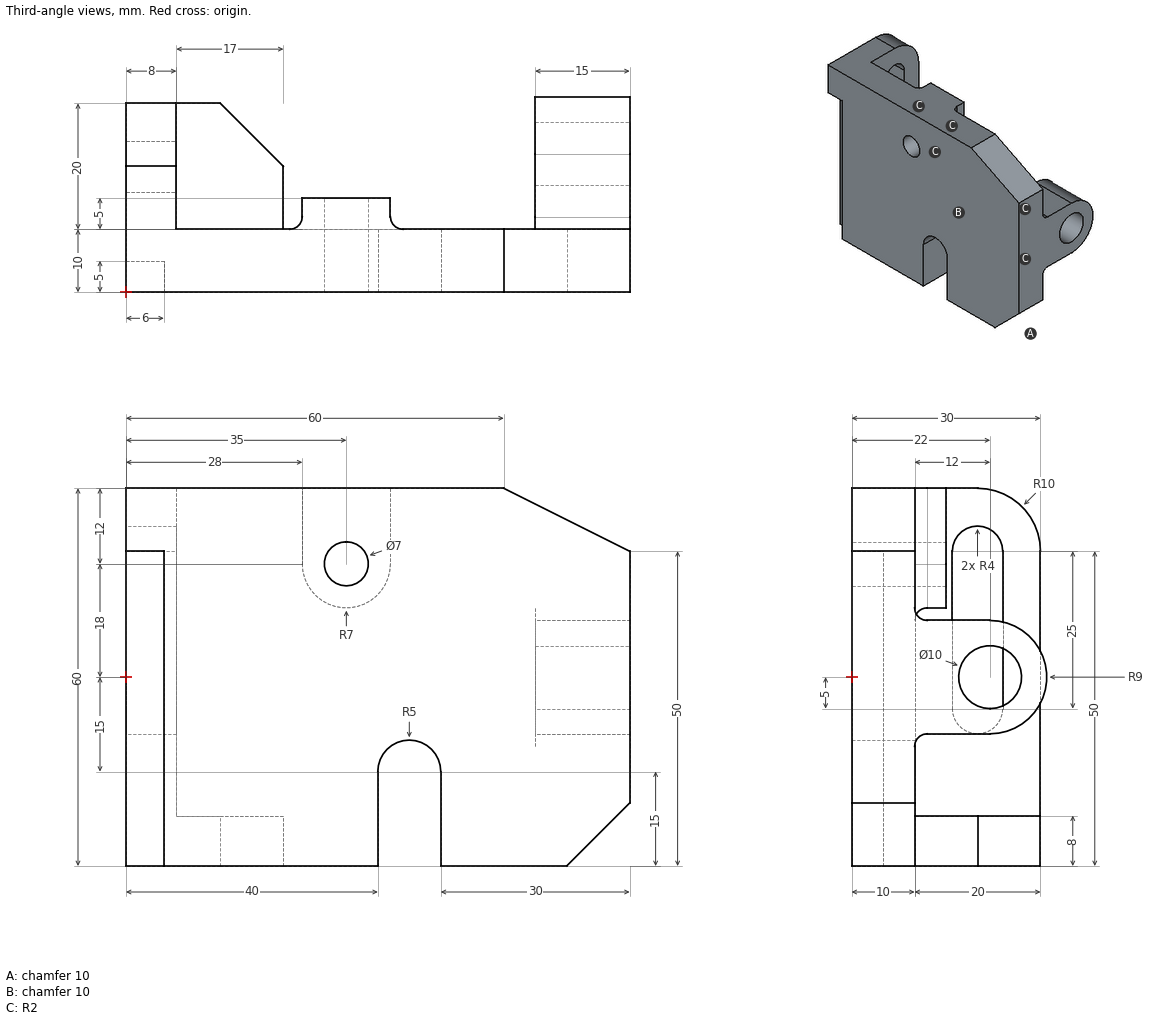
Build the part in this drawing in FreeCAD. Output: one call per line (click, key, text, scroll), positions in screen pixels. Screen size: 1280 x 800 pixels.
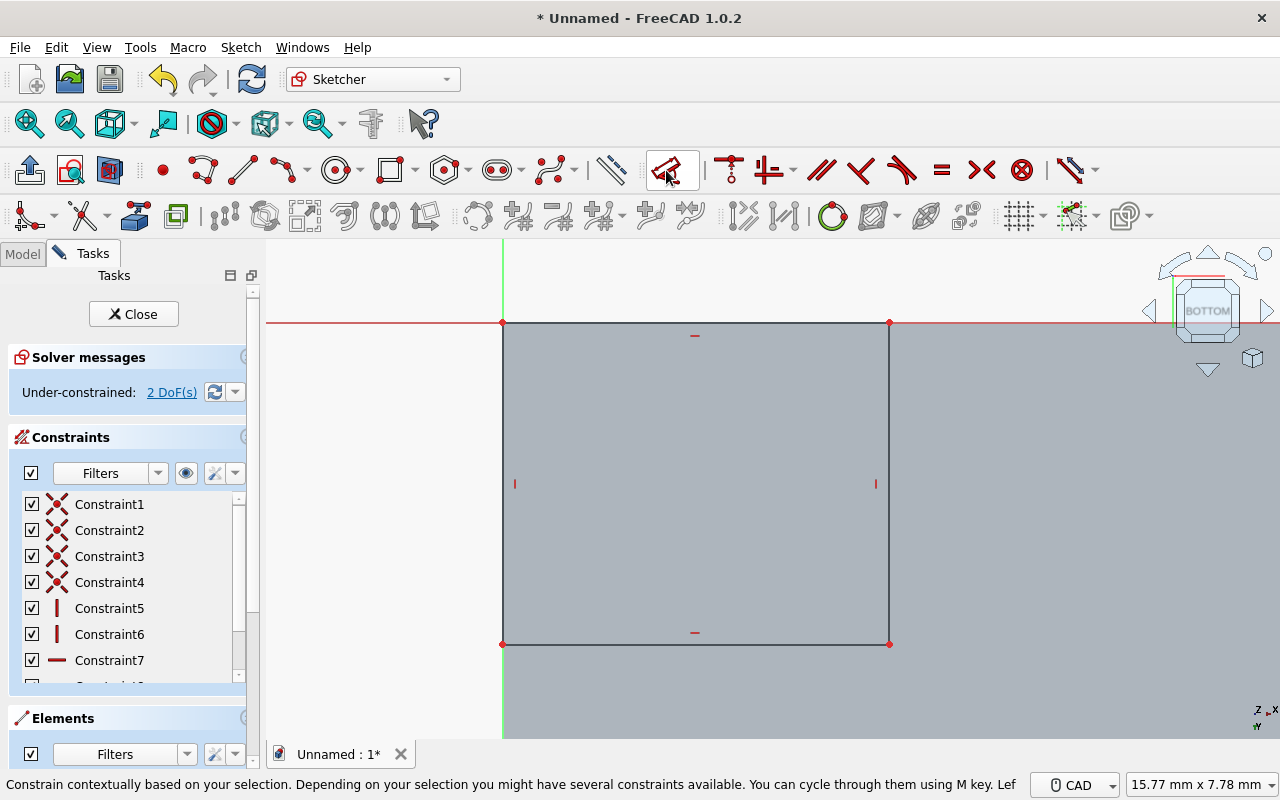
click(503, 419)
click(469, 484)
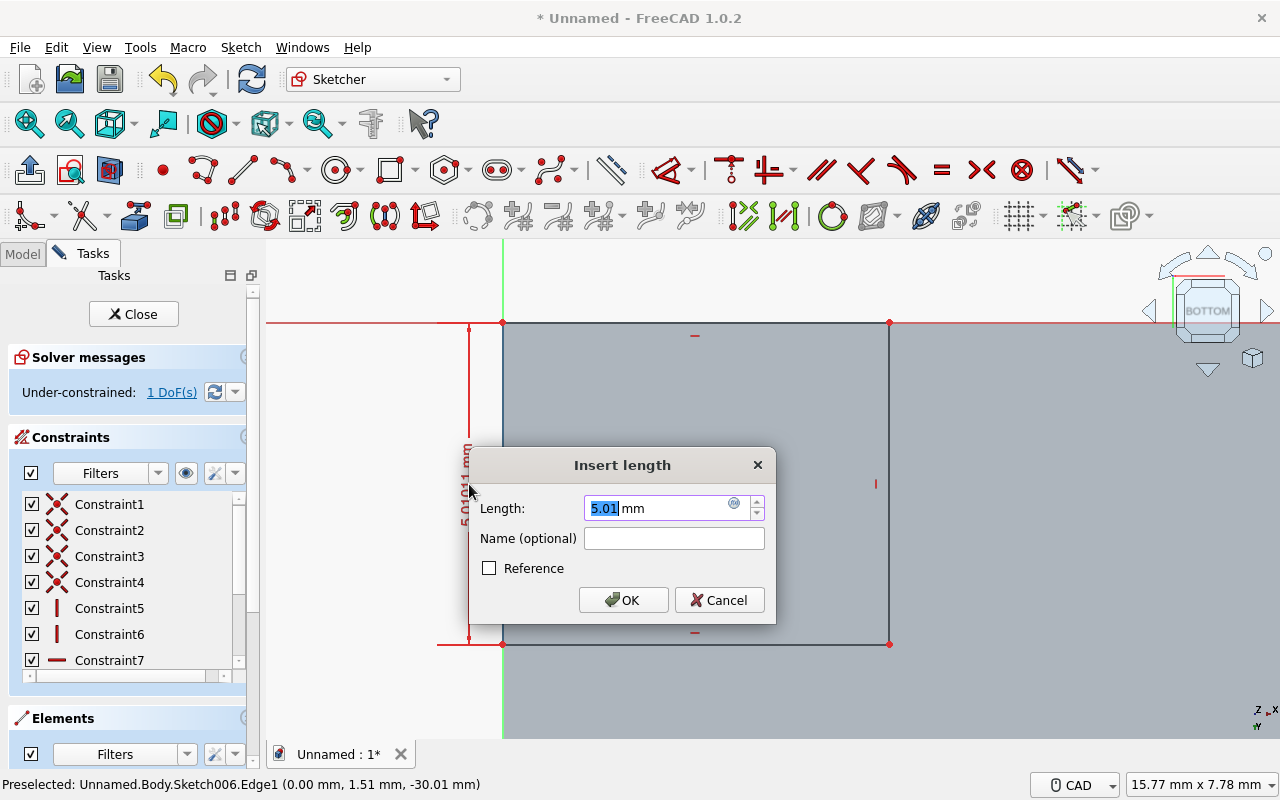
text(5)
key(Return)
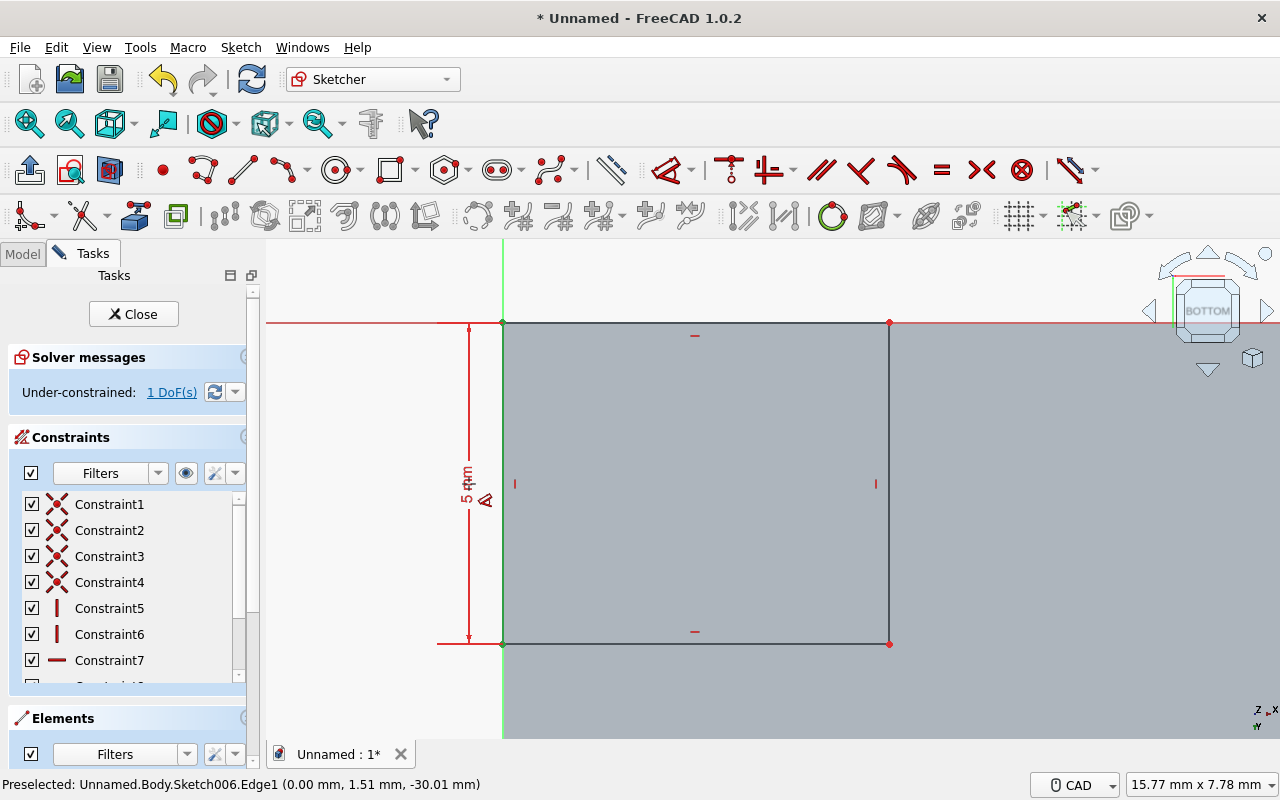
click(619, 644)
click(696, 678)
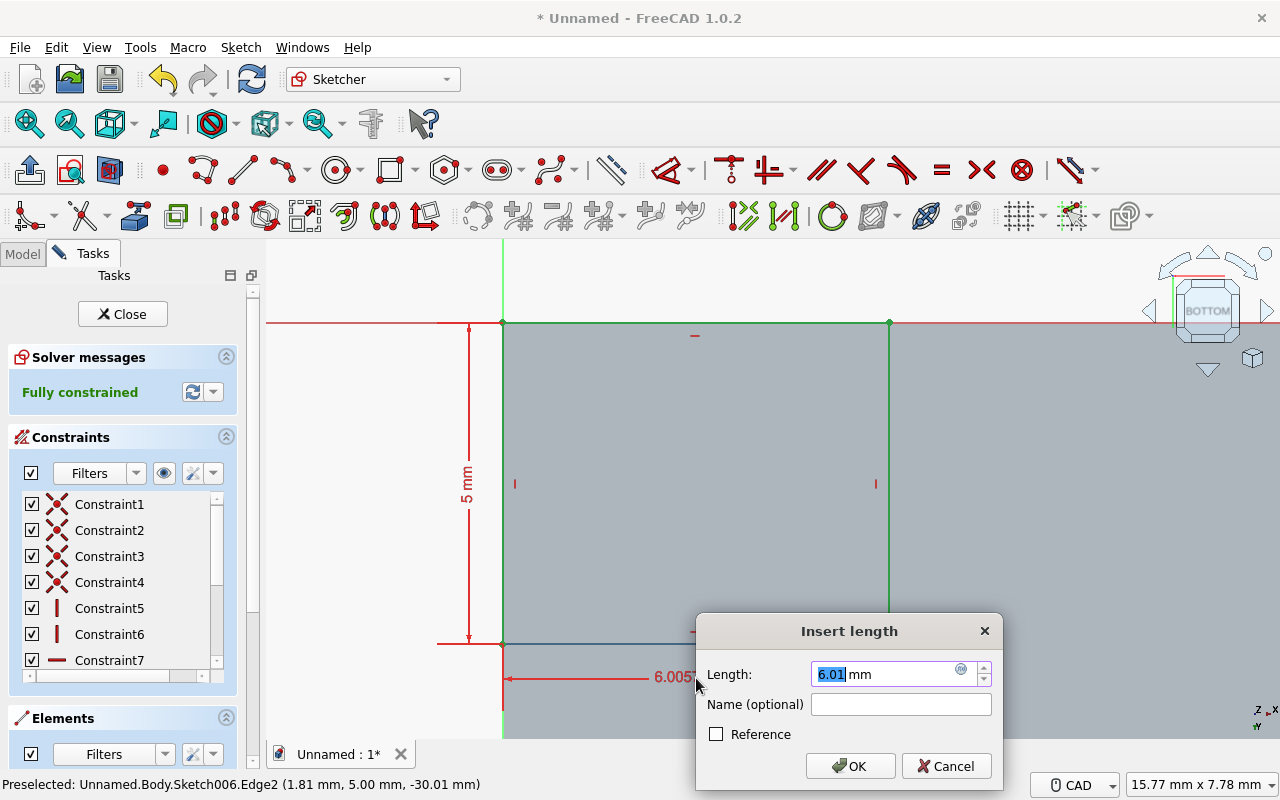
text(6)
key(Return)
key(Escape)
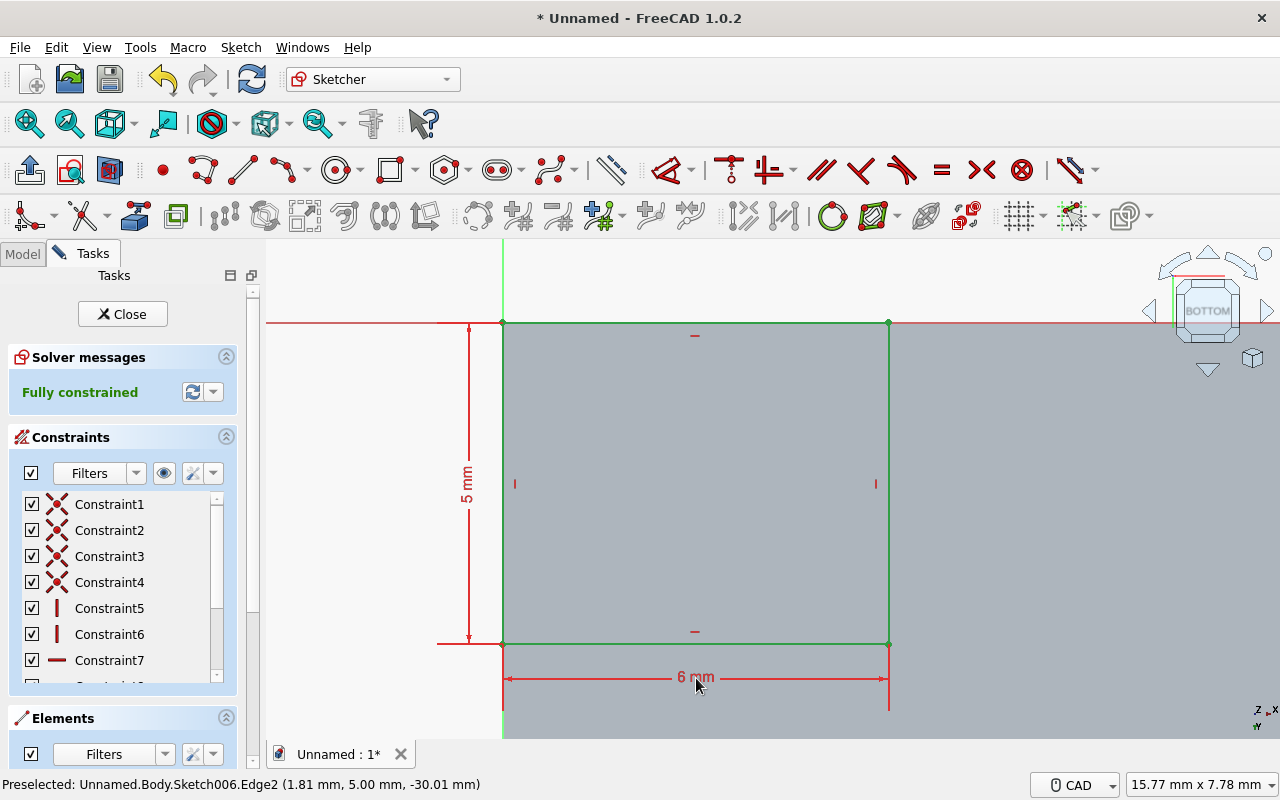
click(123, 314)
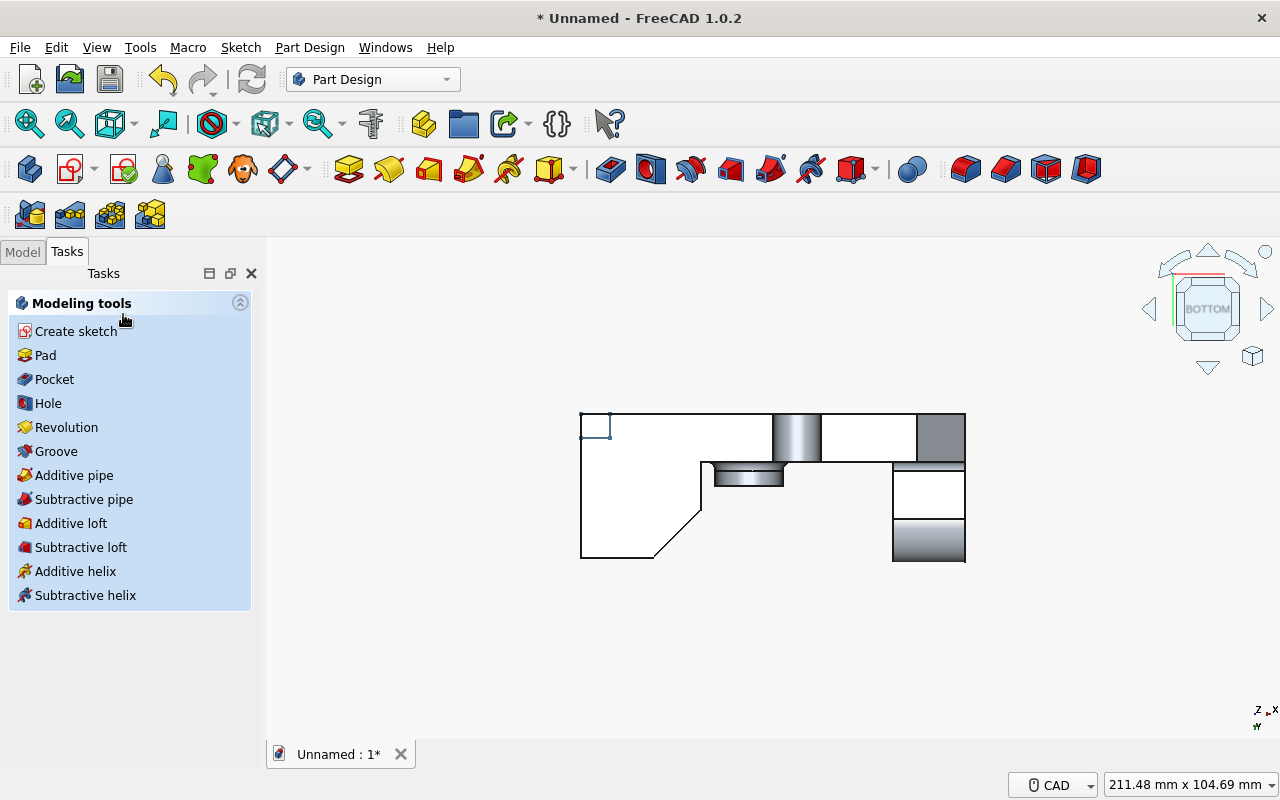
click(612, 170)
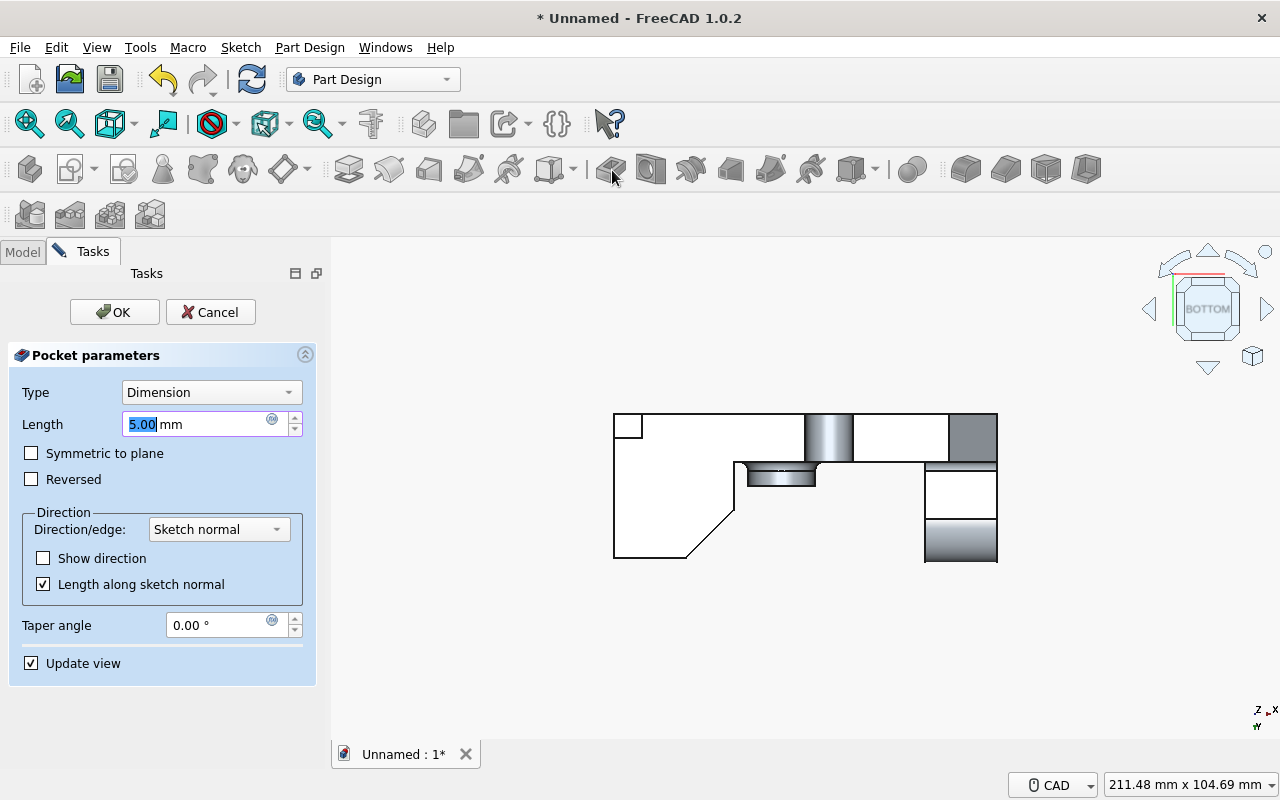
text(50)
key(Tab)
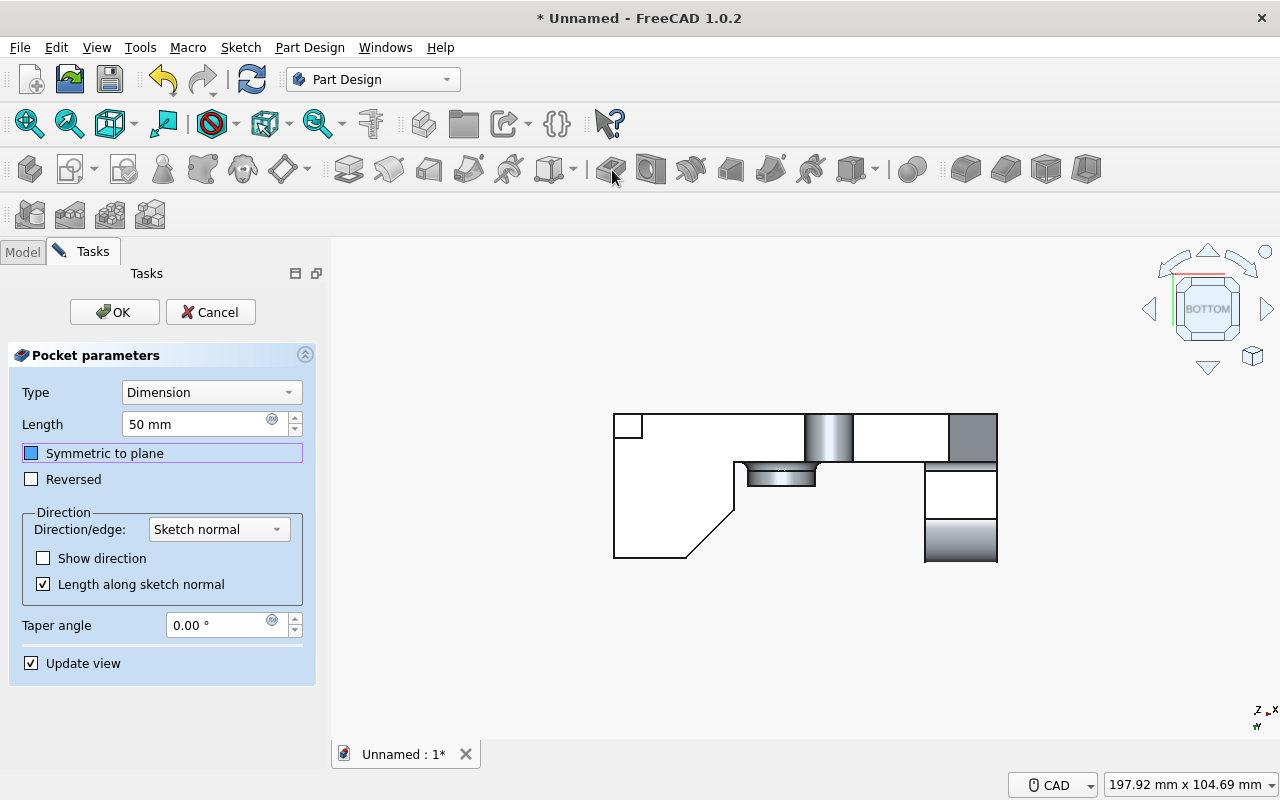
click(115, 312)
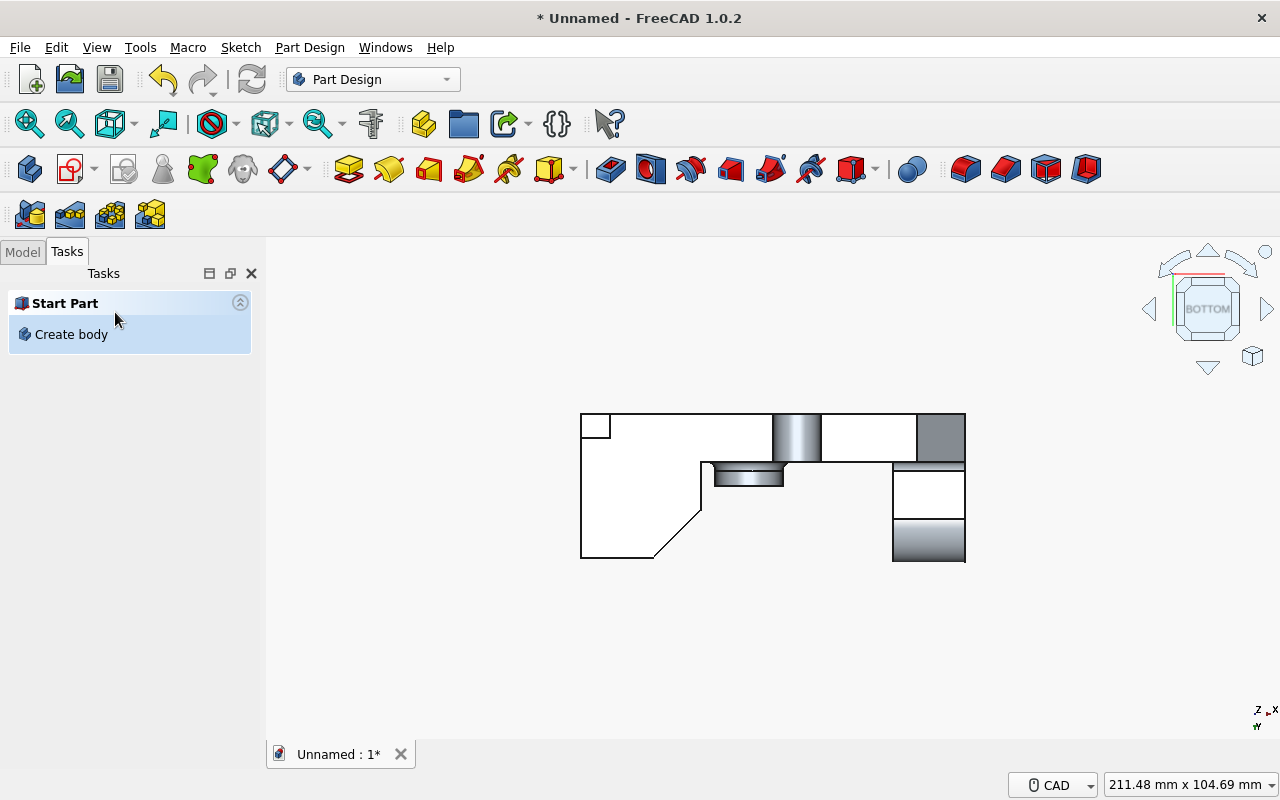
key(0)